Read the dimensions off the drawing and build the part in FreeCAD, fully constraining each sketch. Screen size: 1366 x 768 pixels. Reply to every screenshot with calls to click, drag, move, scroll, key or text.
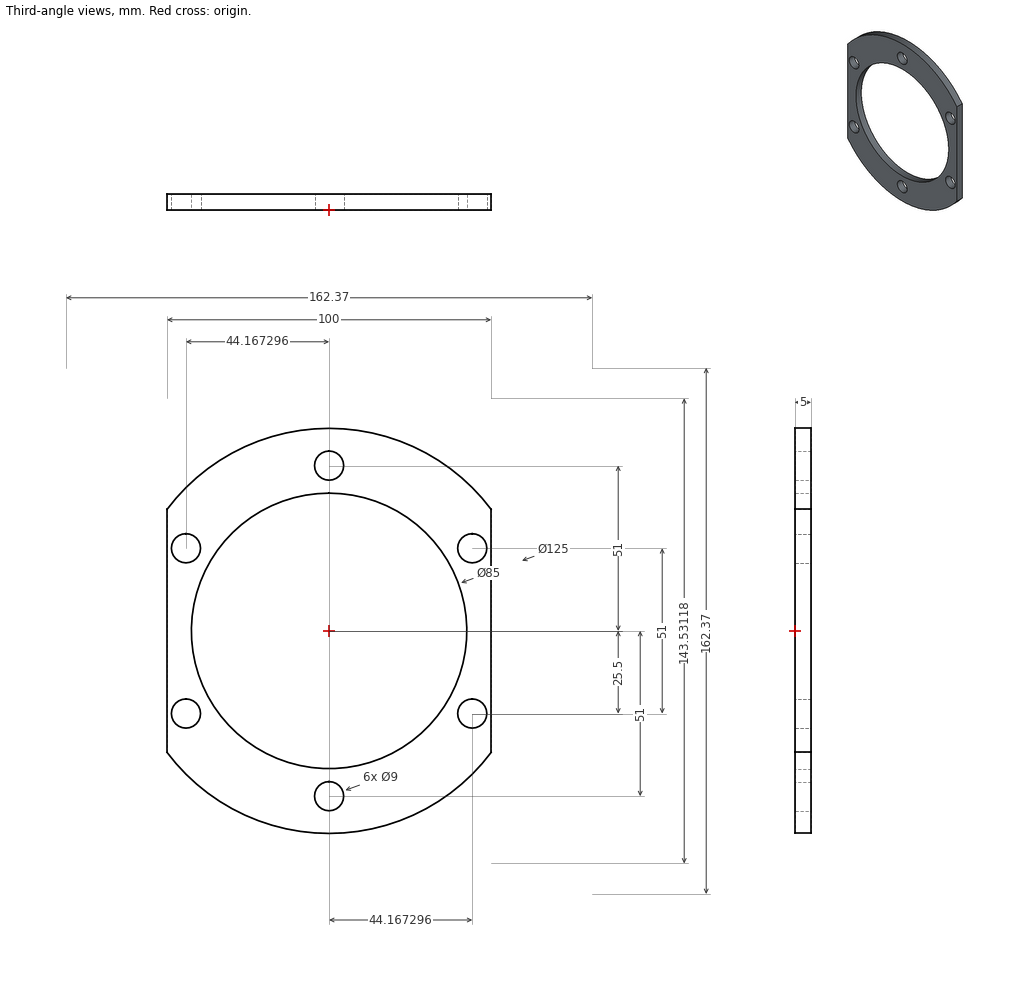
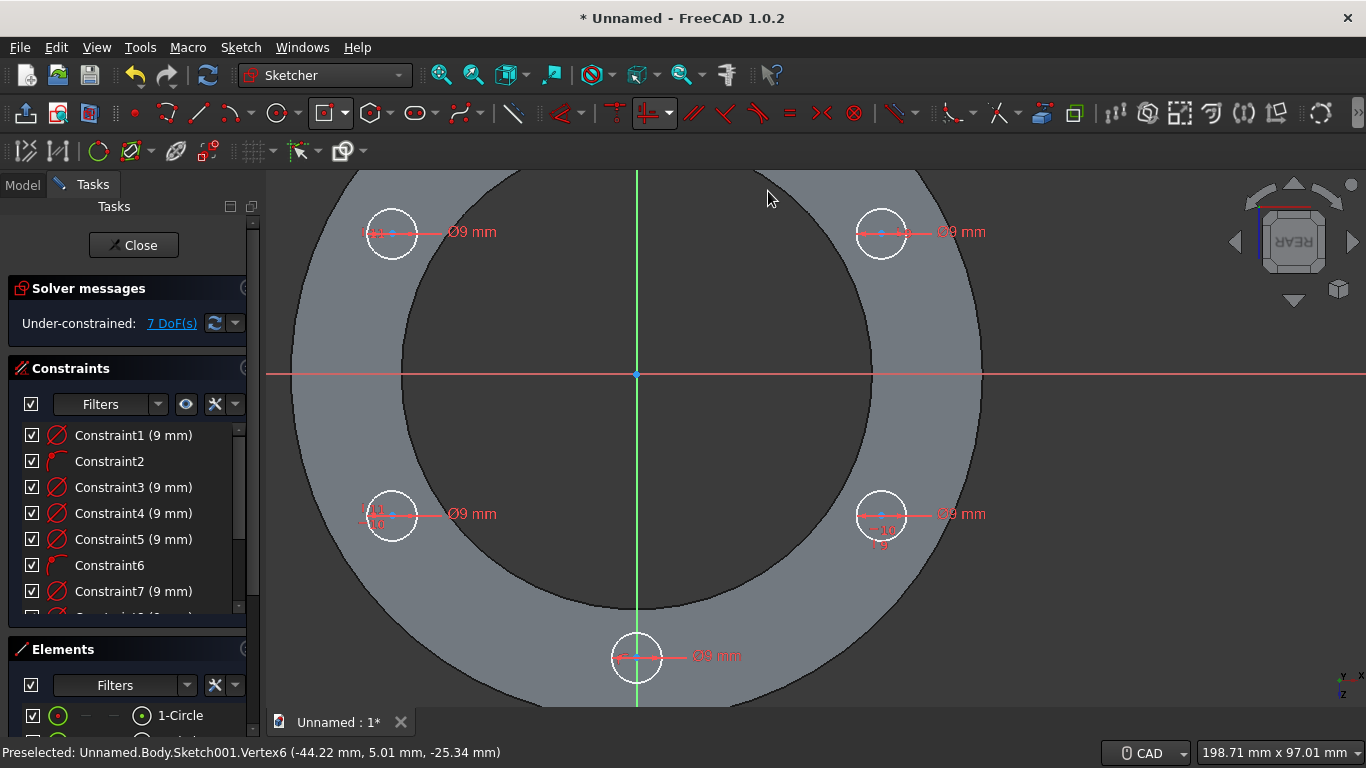
click(881, 234)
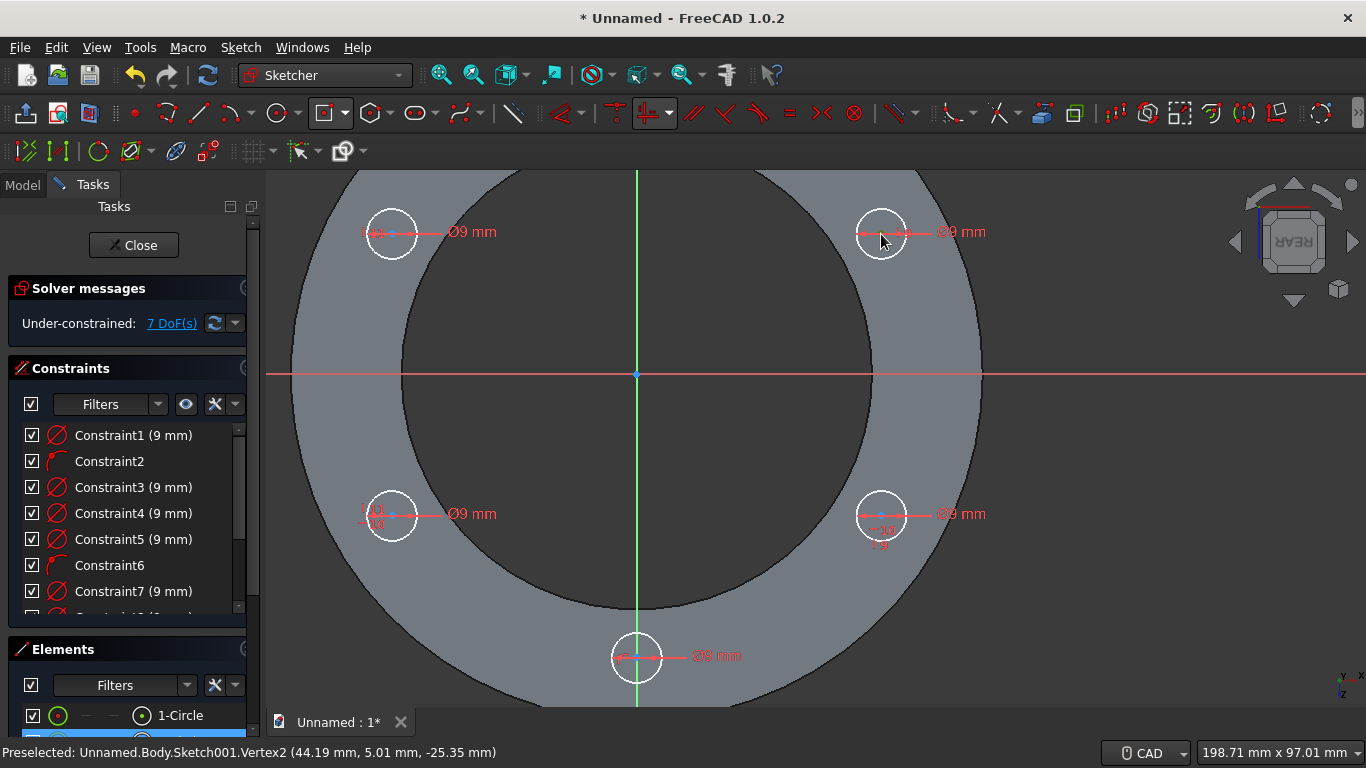
click(392, 234)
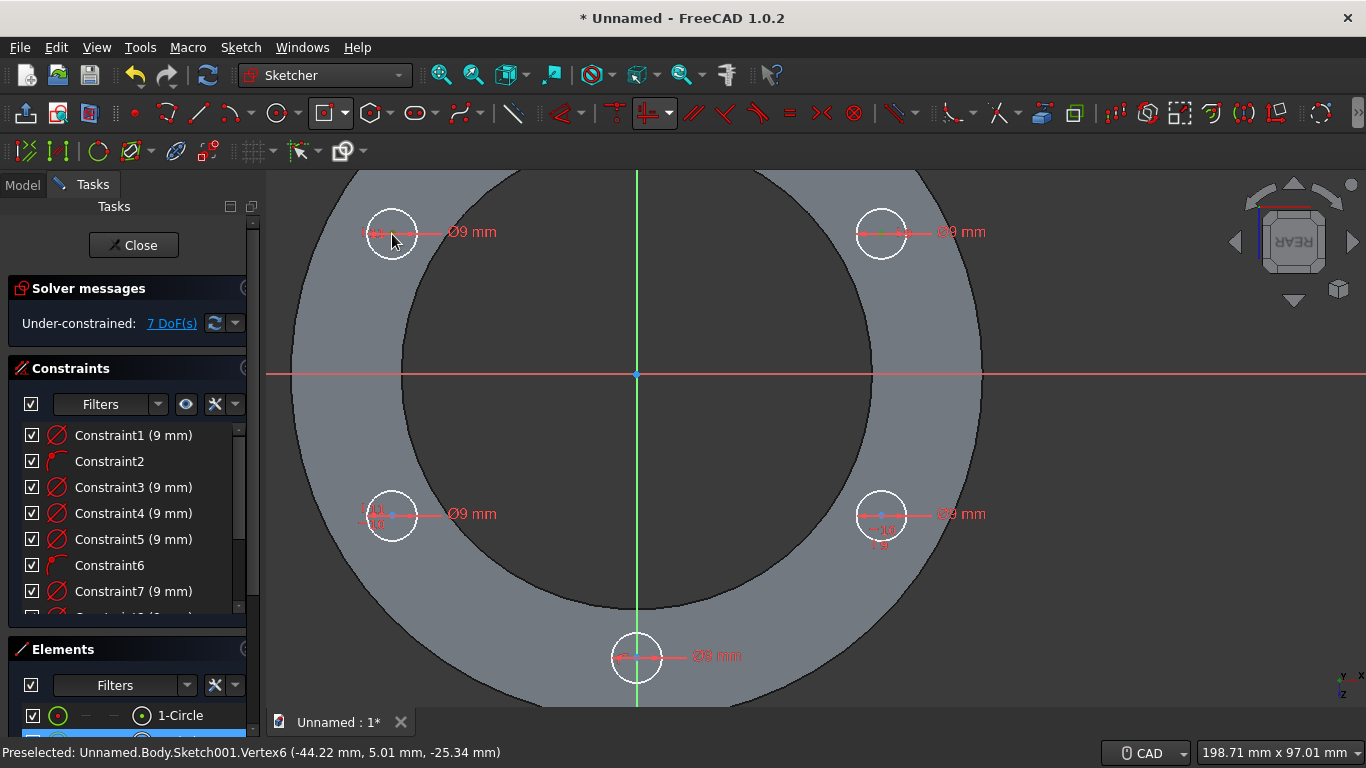
click(672, 114)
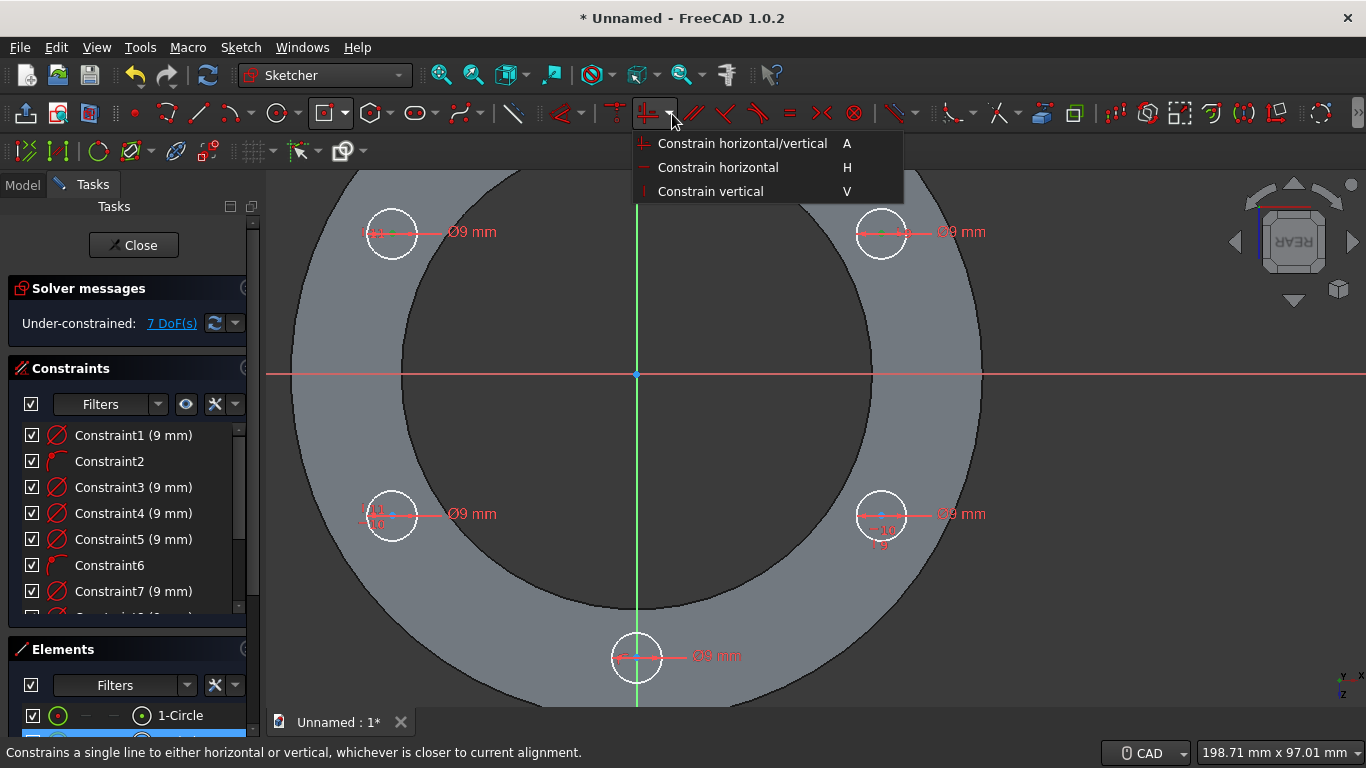
click(768, 167)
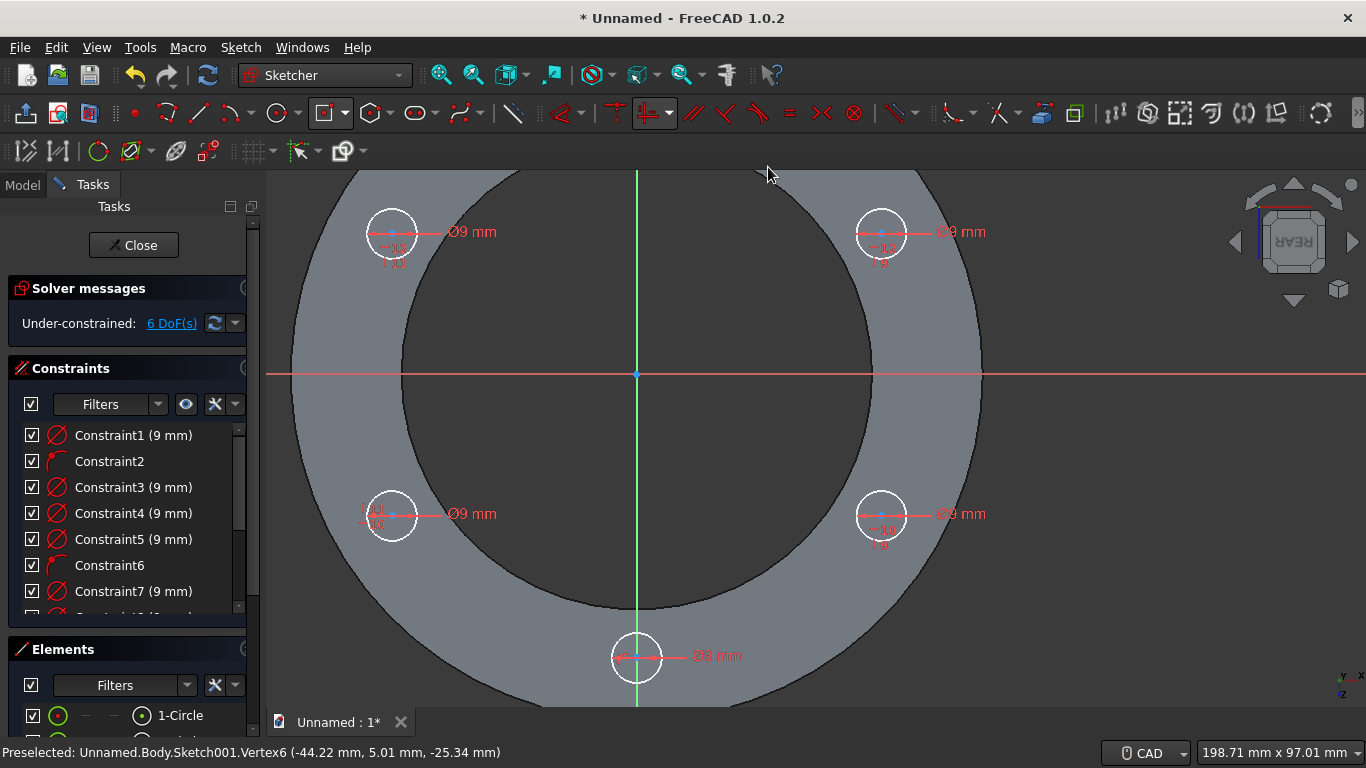
scroll(882, 517, down, 3)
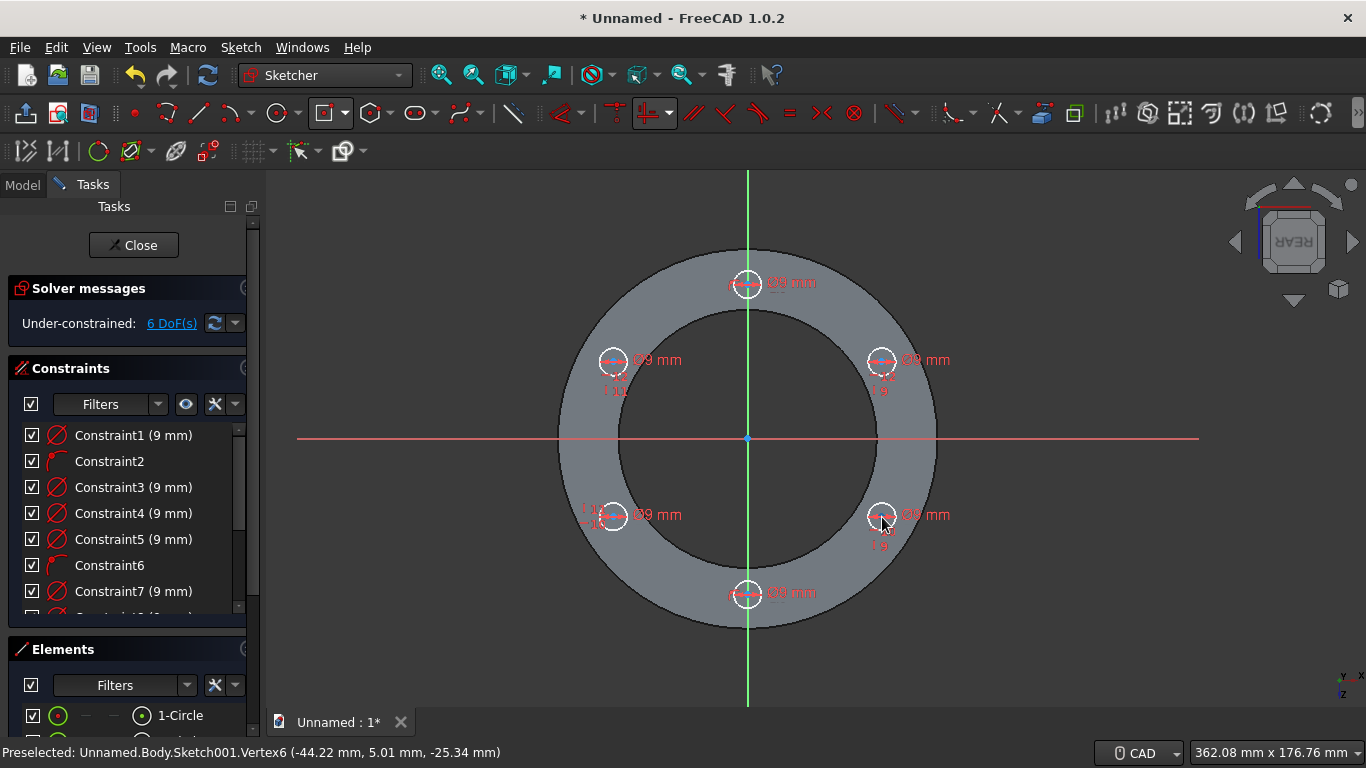
click(748, 285)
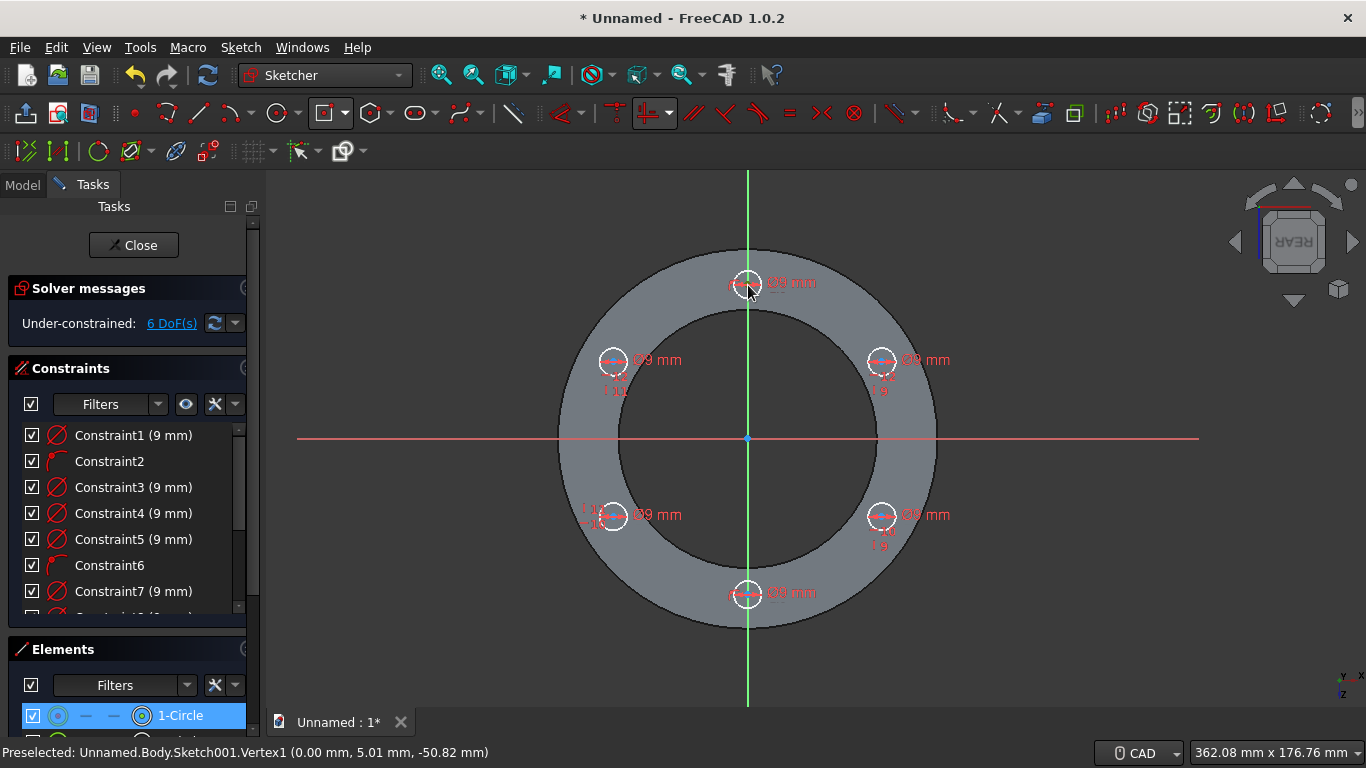
click(584, 114)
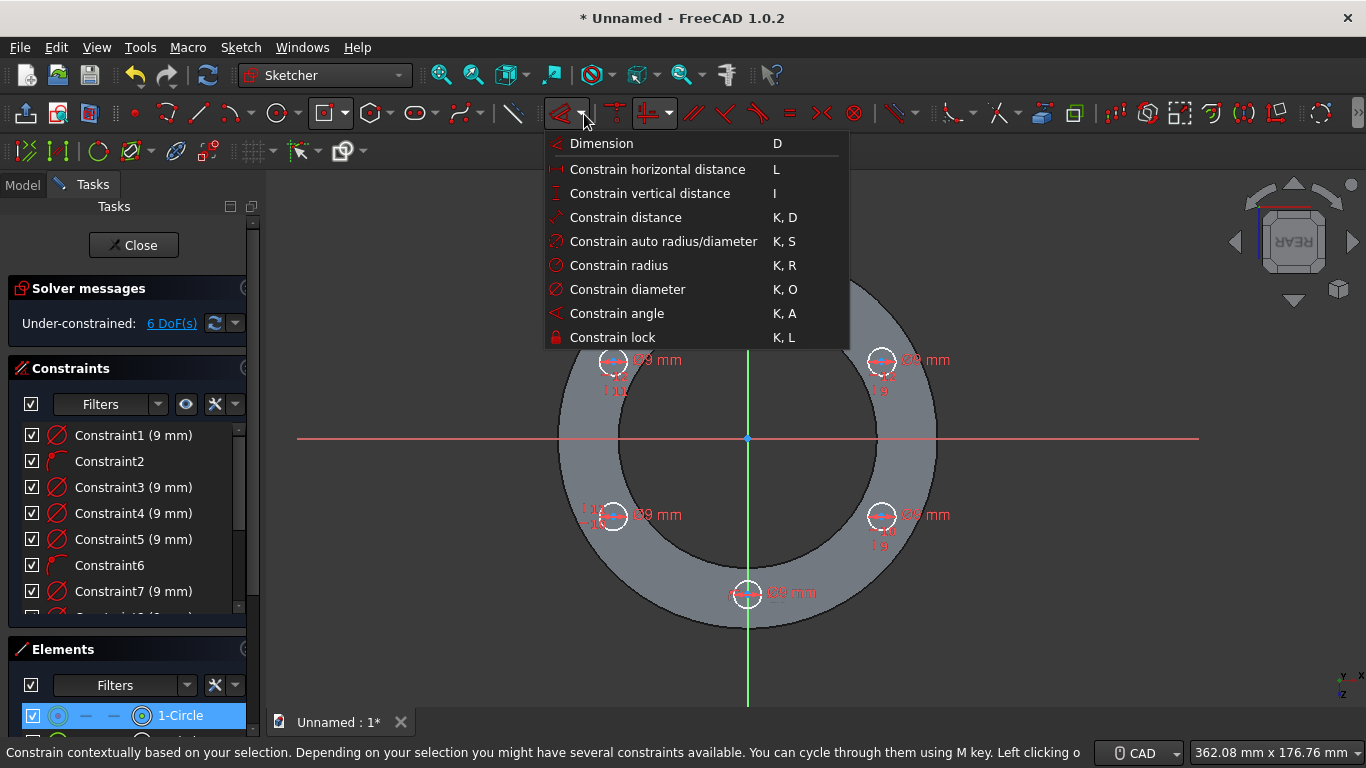
click(697, 193)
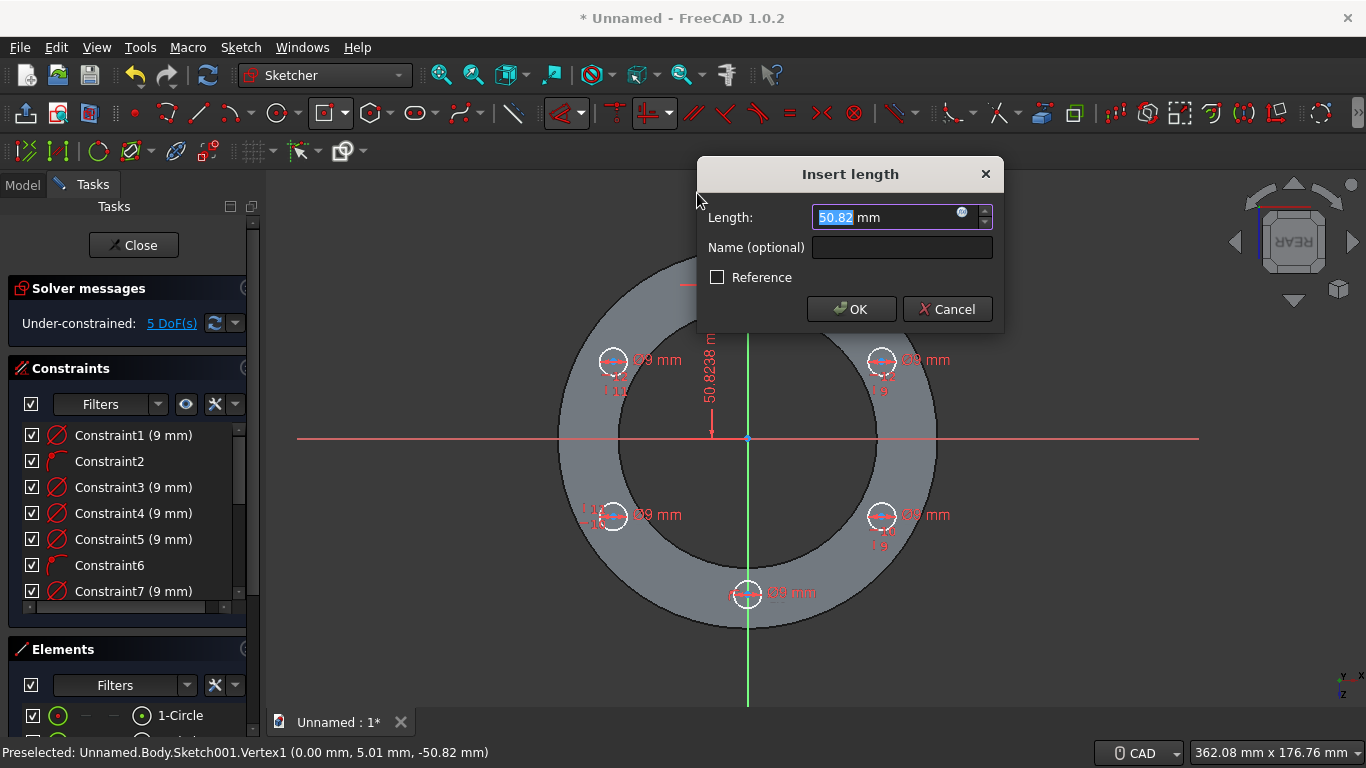
text(51)
key(Return)